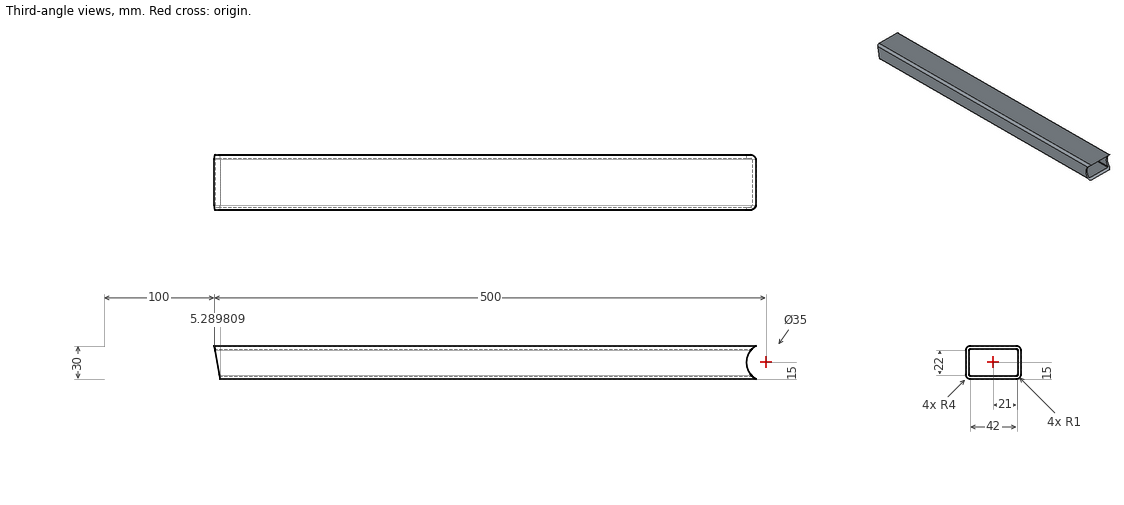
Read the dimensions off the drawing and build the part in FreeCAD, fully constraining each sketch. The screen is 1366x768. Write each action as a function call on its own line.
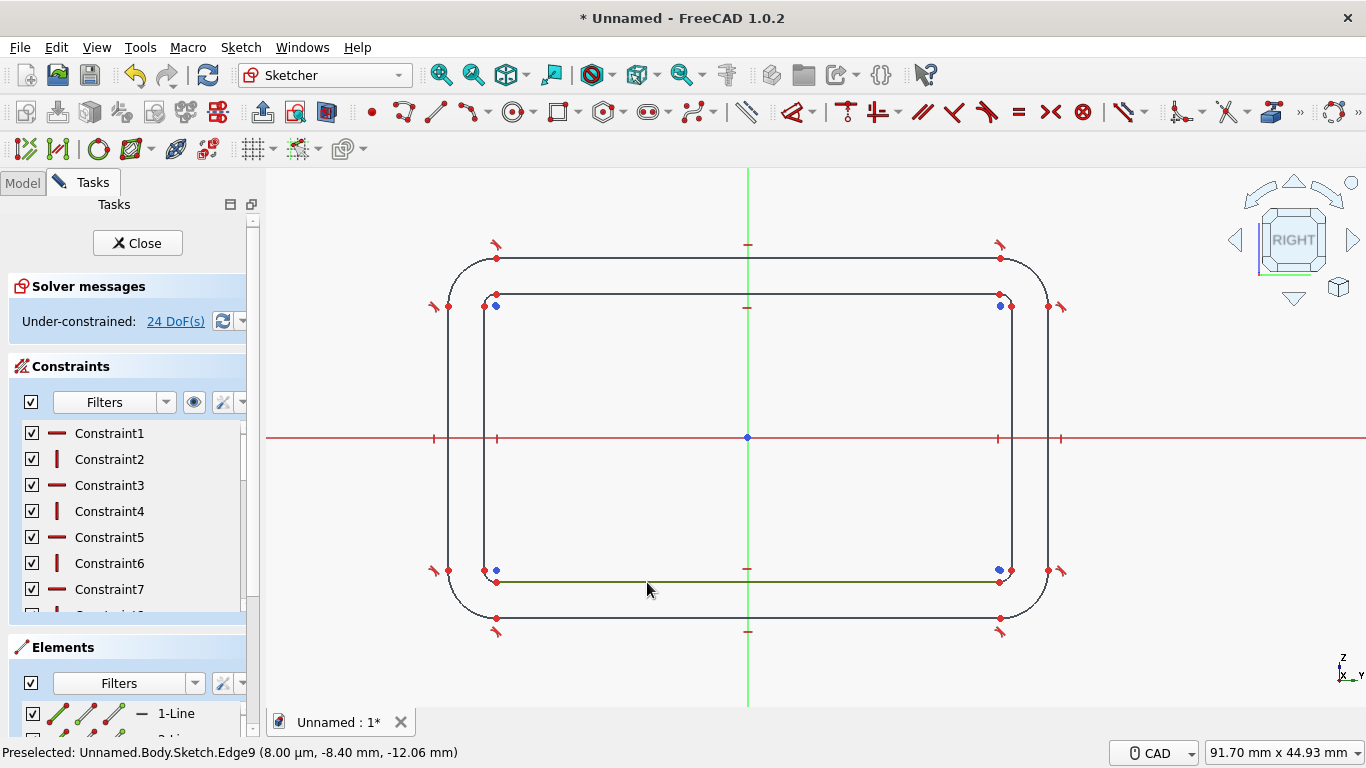
scroll(1008, 579, up, 3)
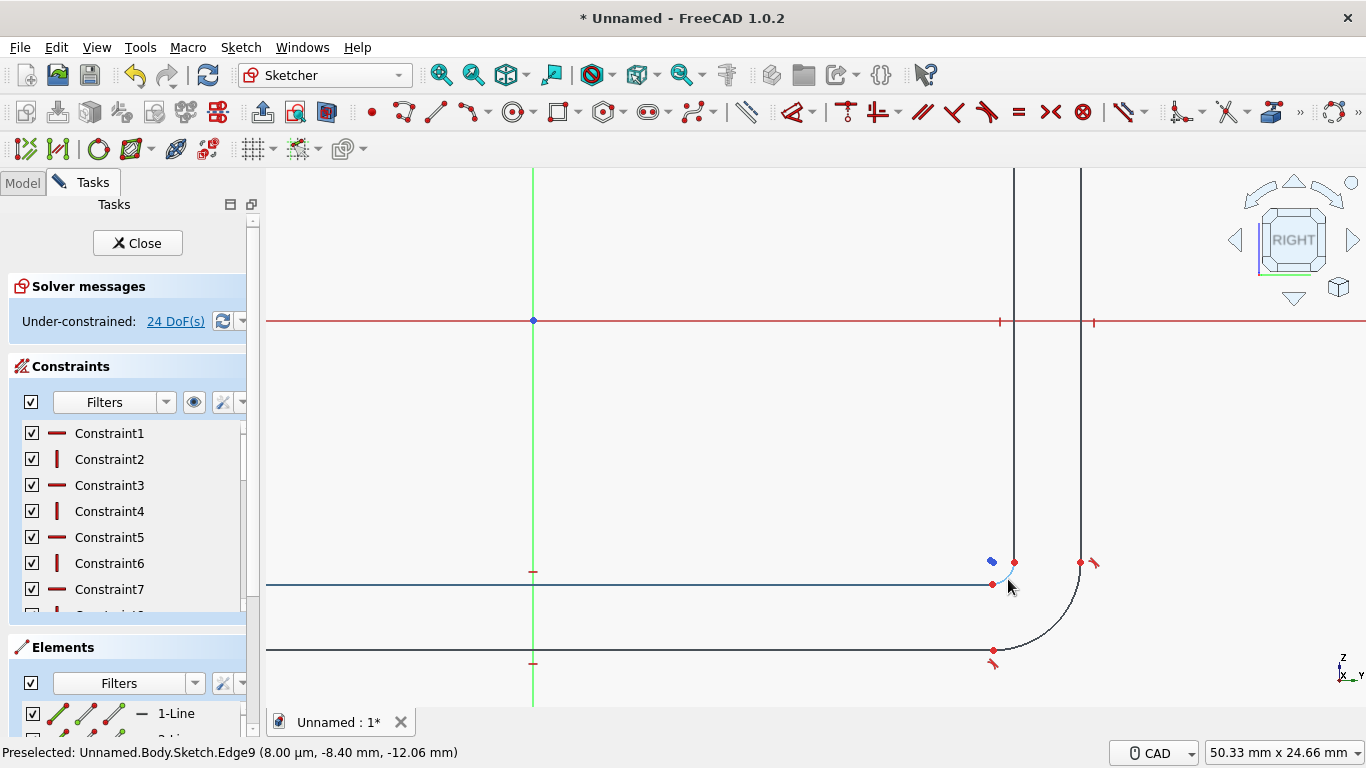
click(1007, 578)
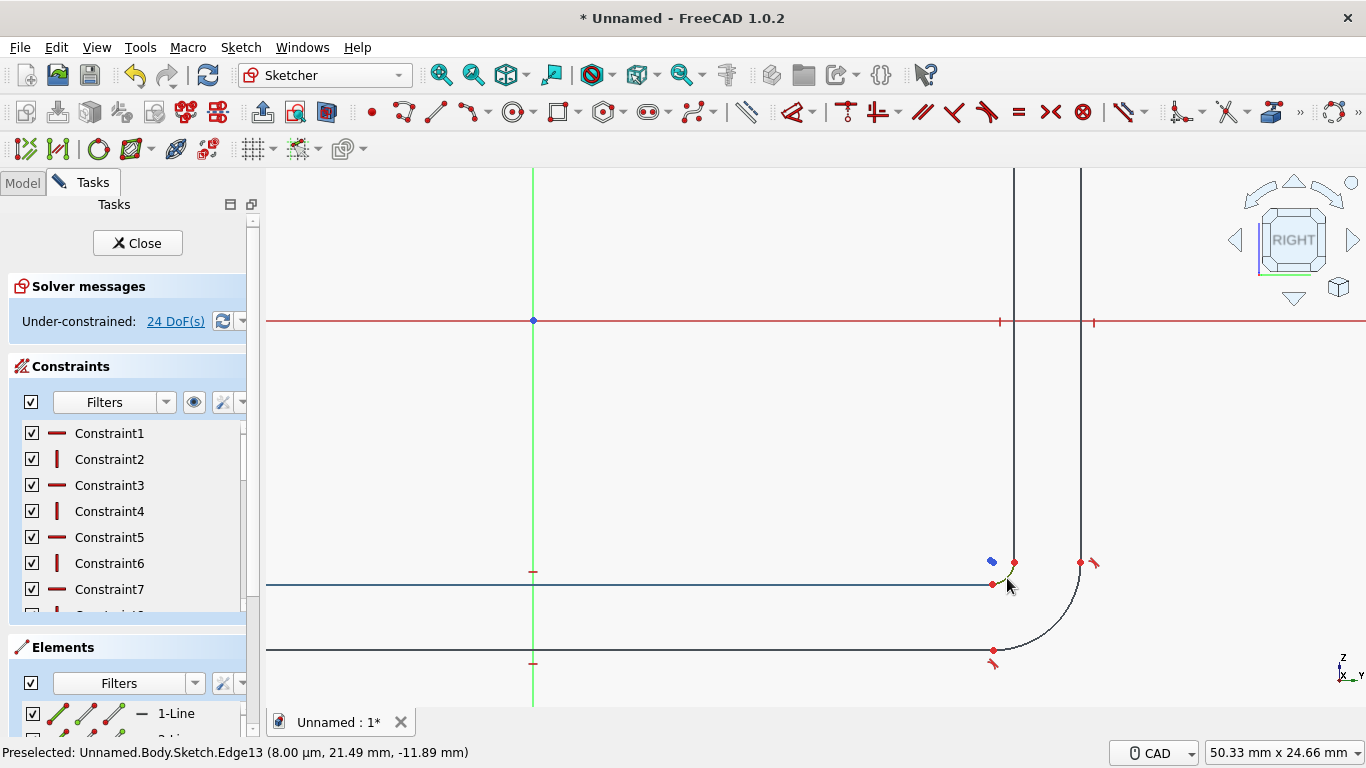
key(t)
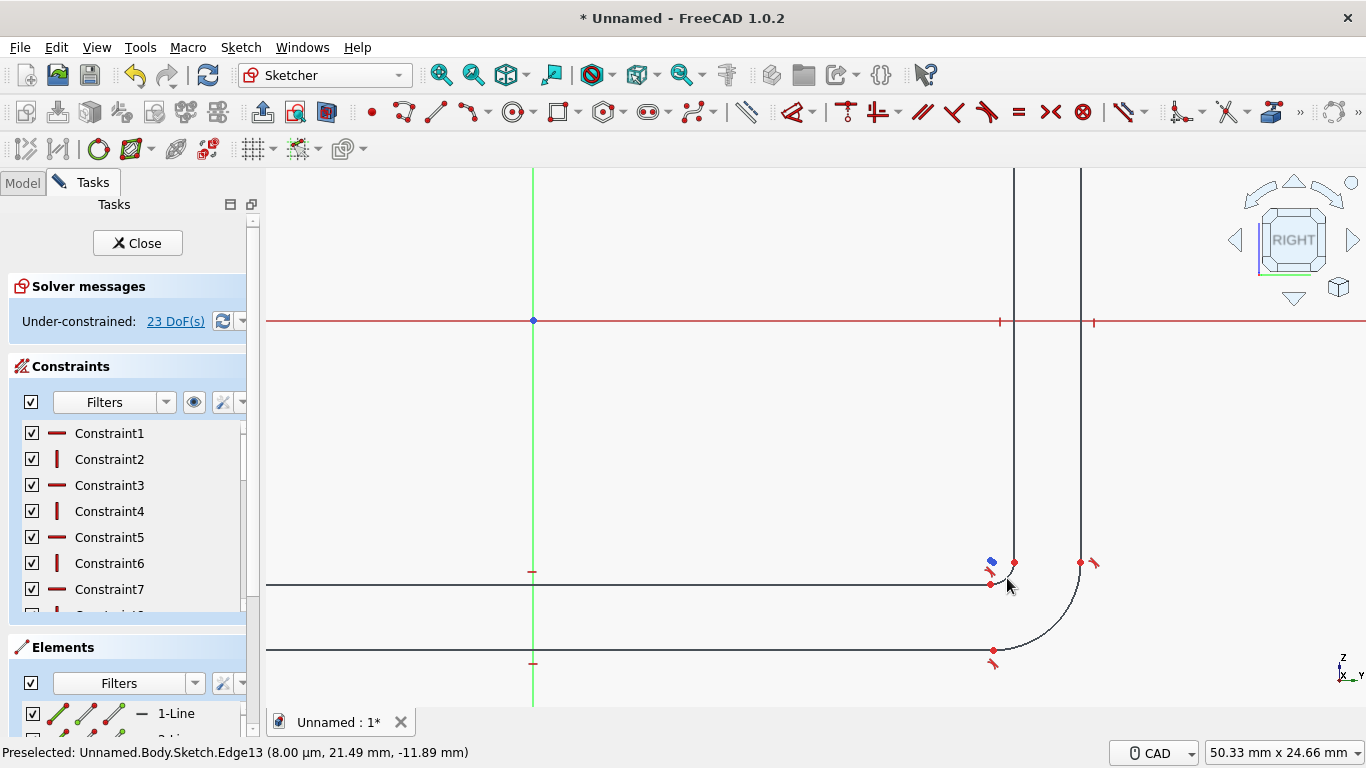
click(349, 585)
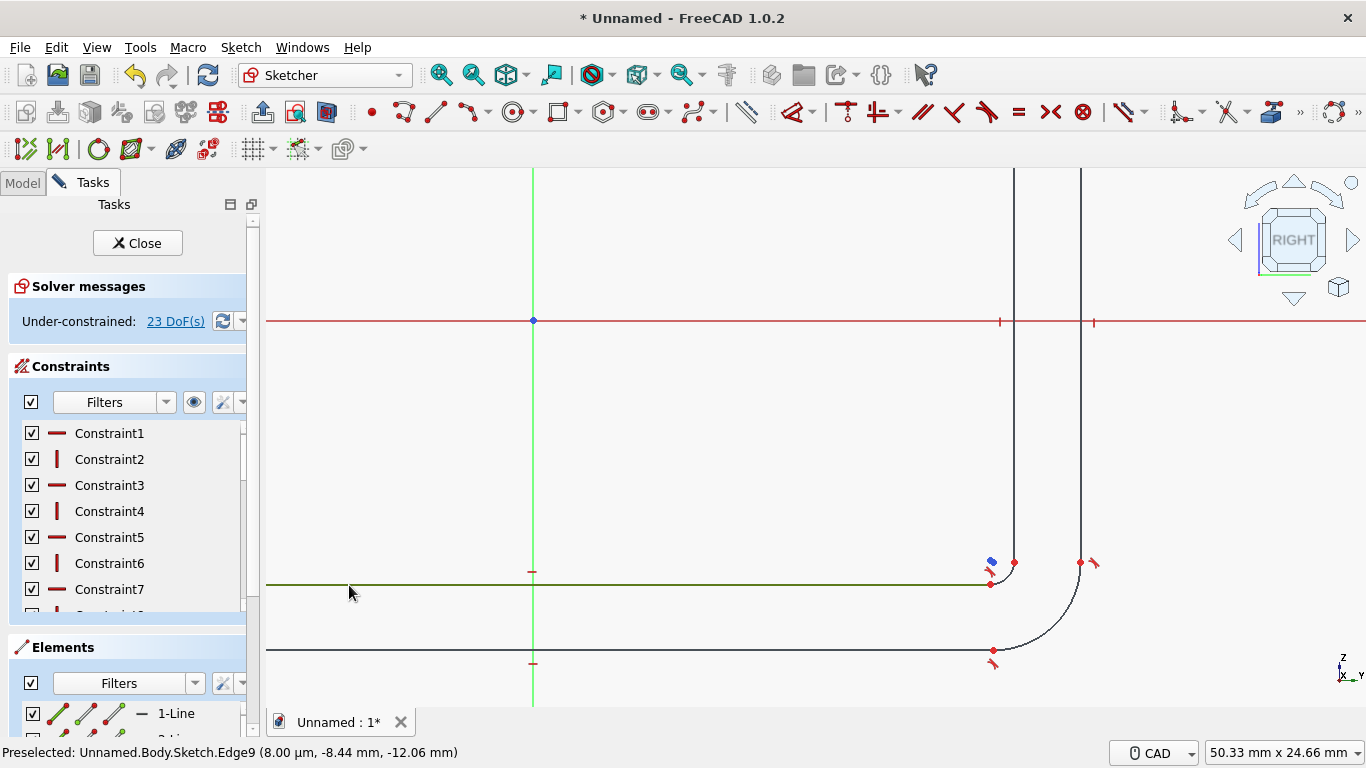
scroll(1008, 579, down, 3)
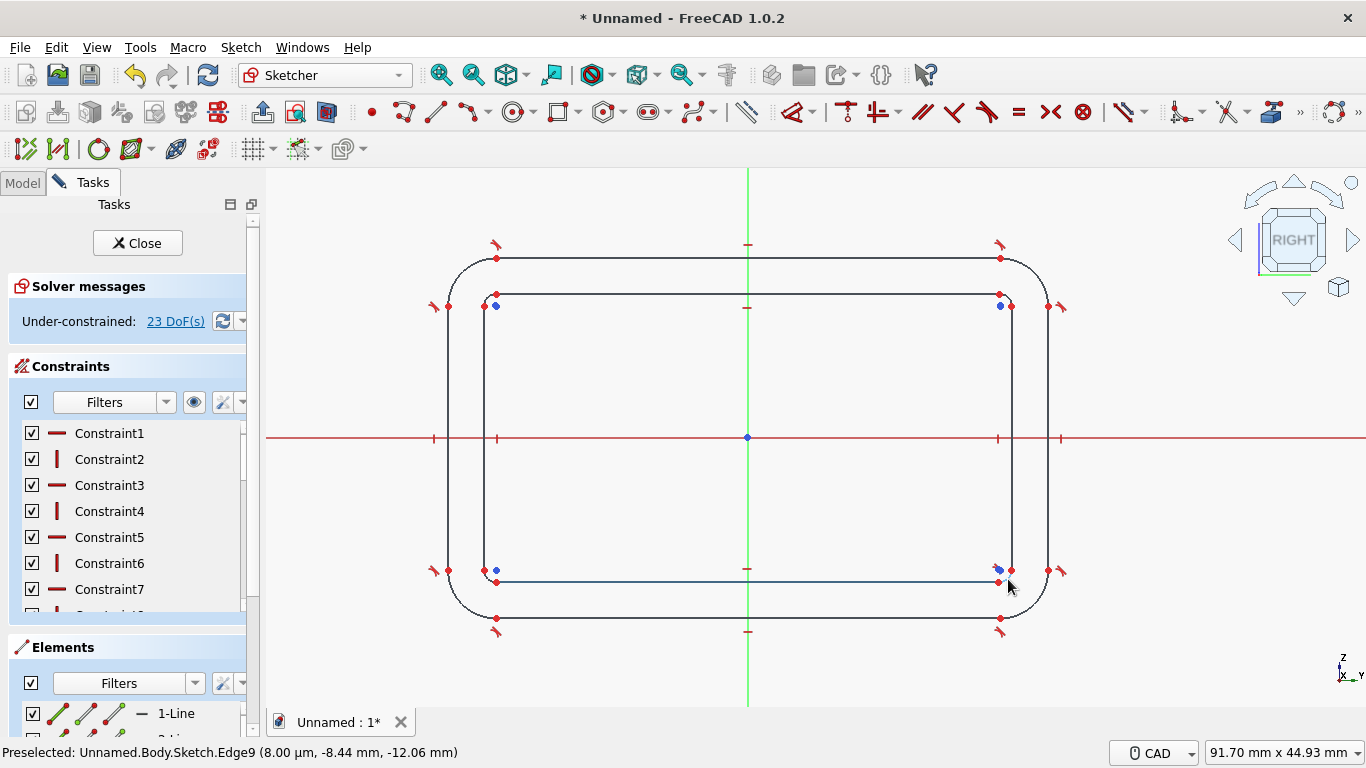
scroll(486, 576, up, 5)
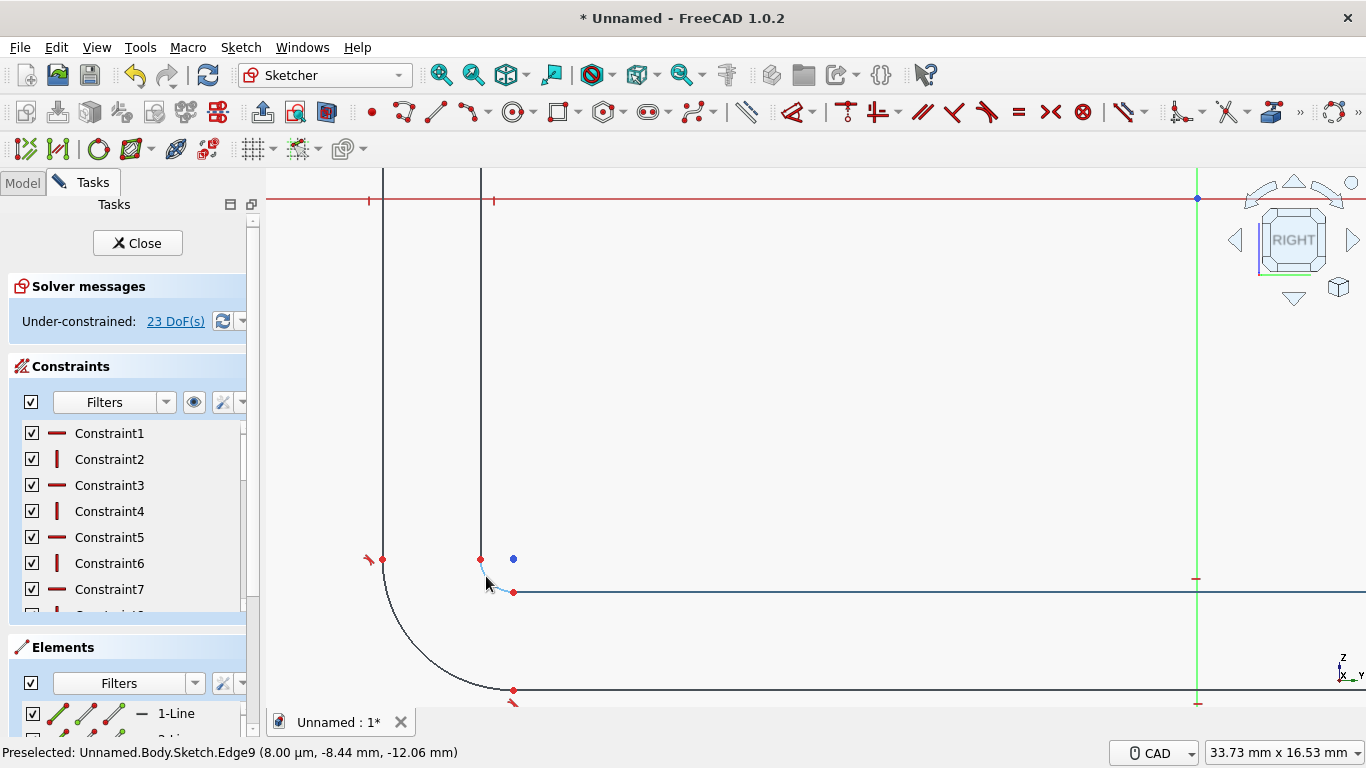
click(484, 574)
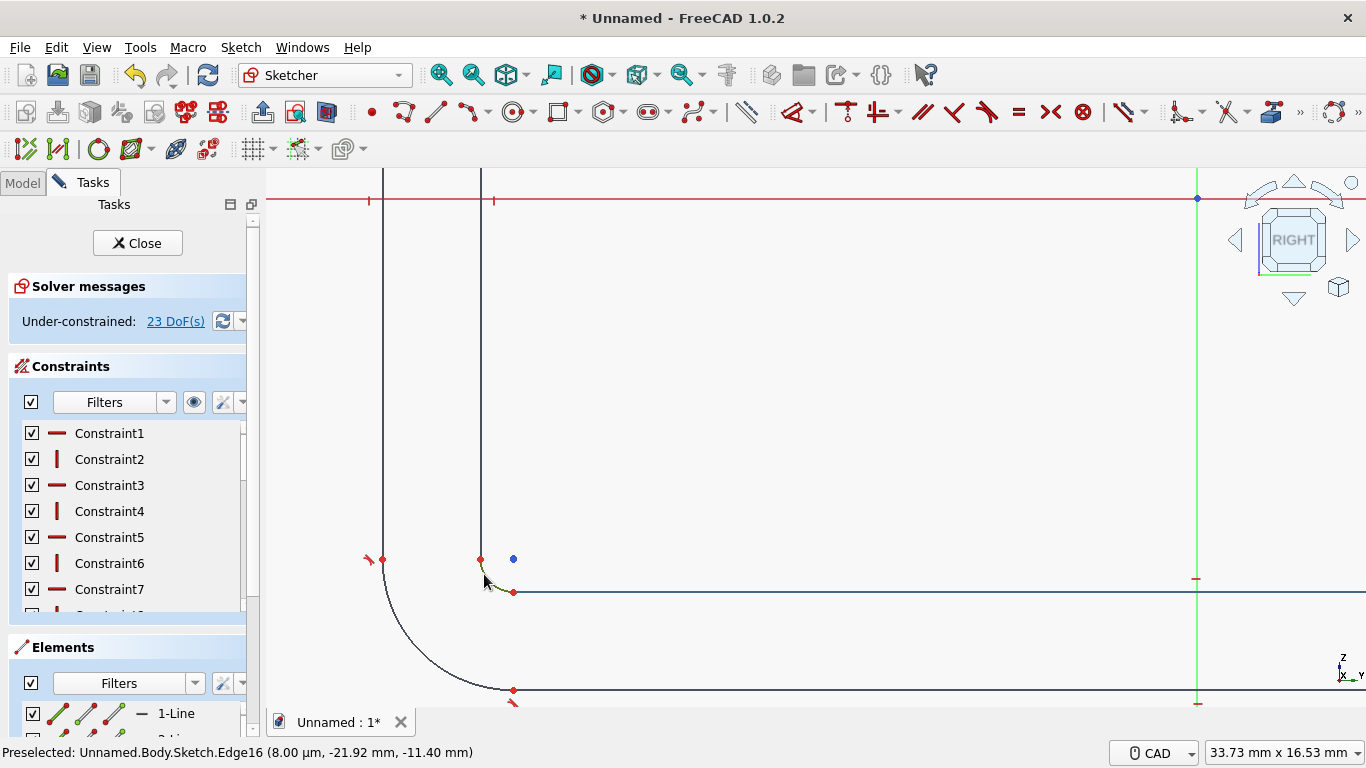
key(t)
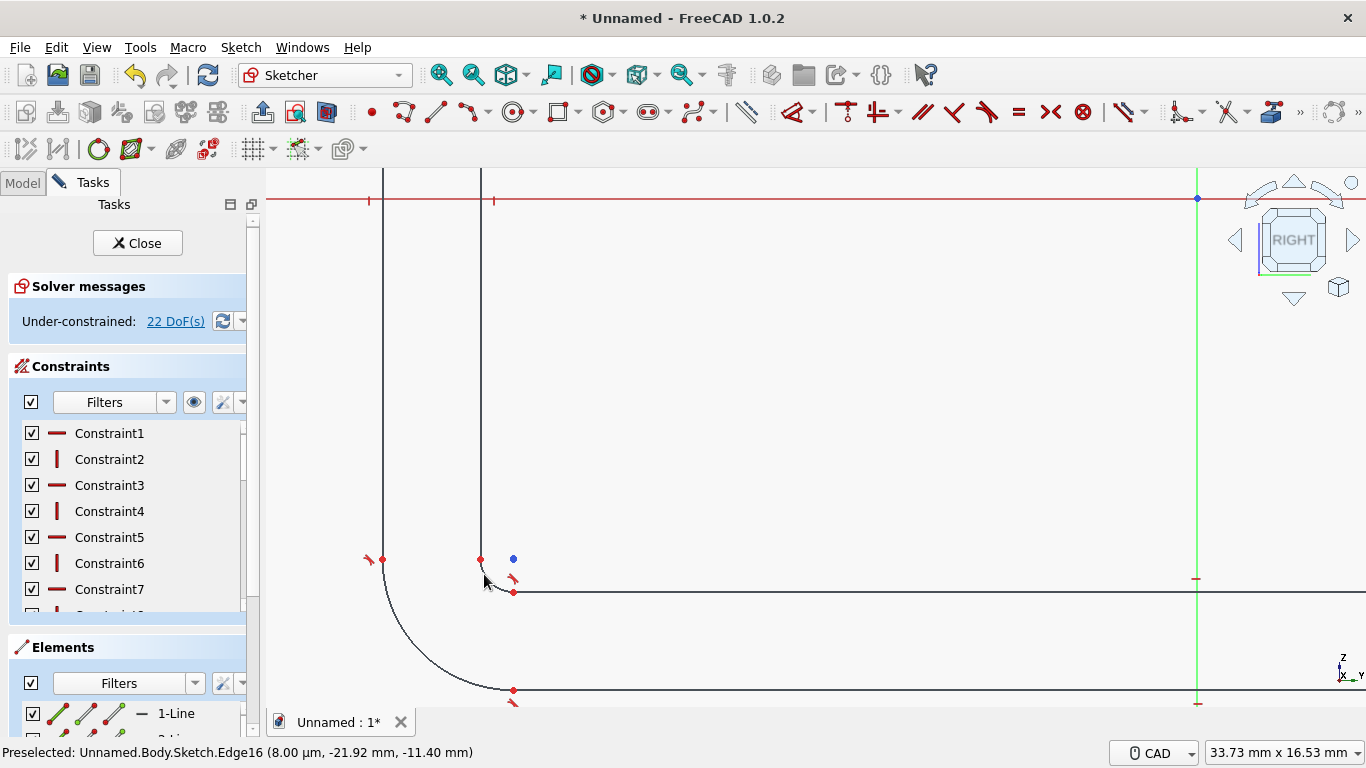
scroll(486, 576, down, 5)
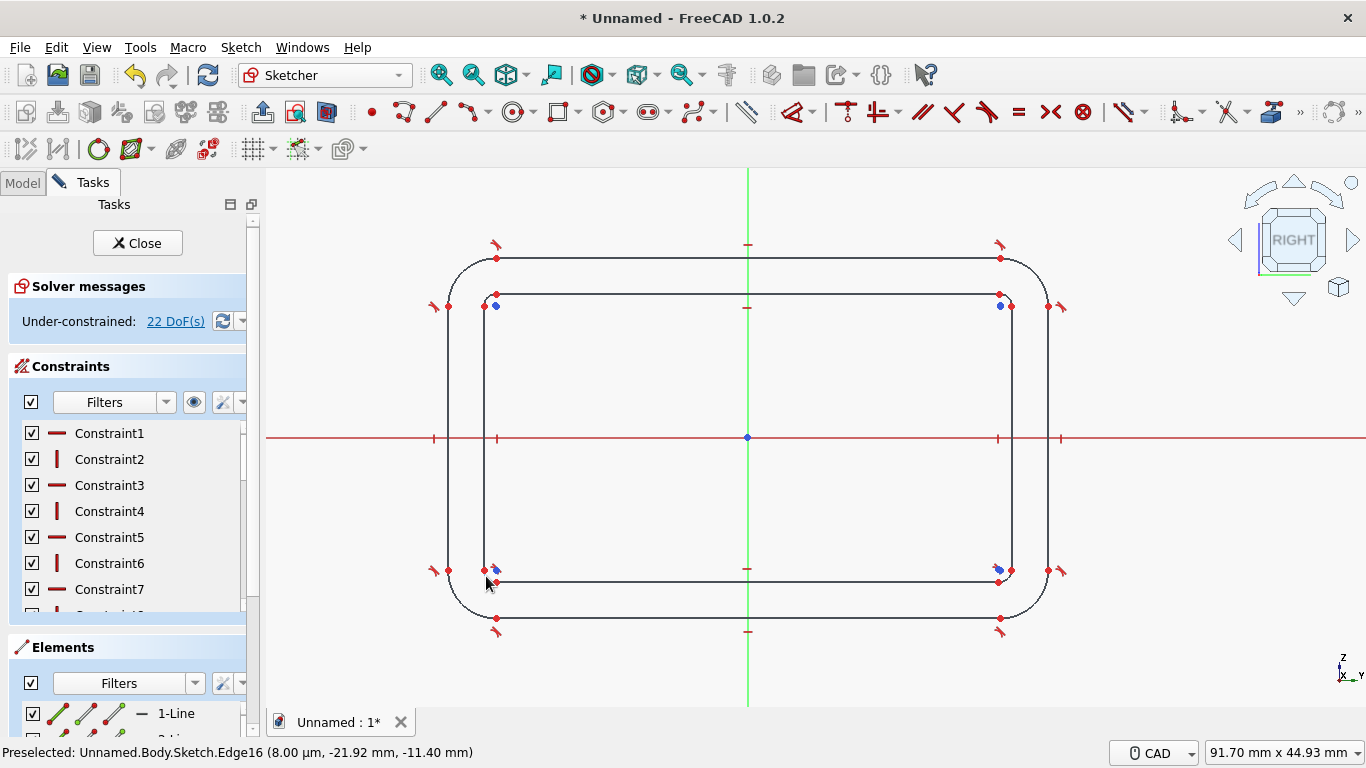
click(1012, 491)